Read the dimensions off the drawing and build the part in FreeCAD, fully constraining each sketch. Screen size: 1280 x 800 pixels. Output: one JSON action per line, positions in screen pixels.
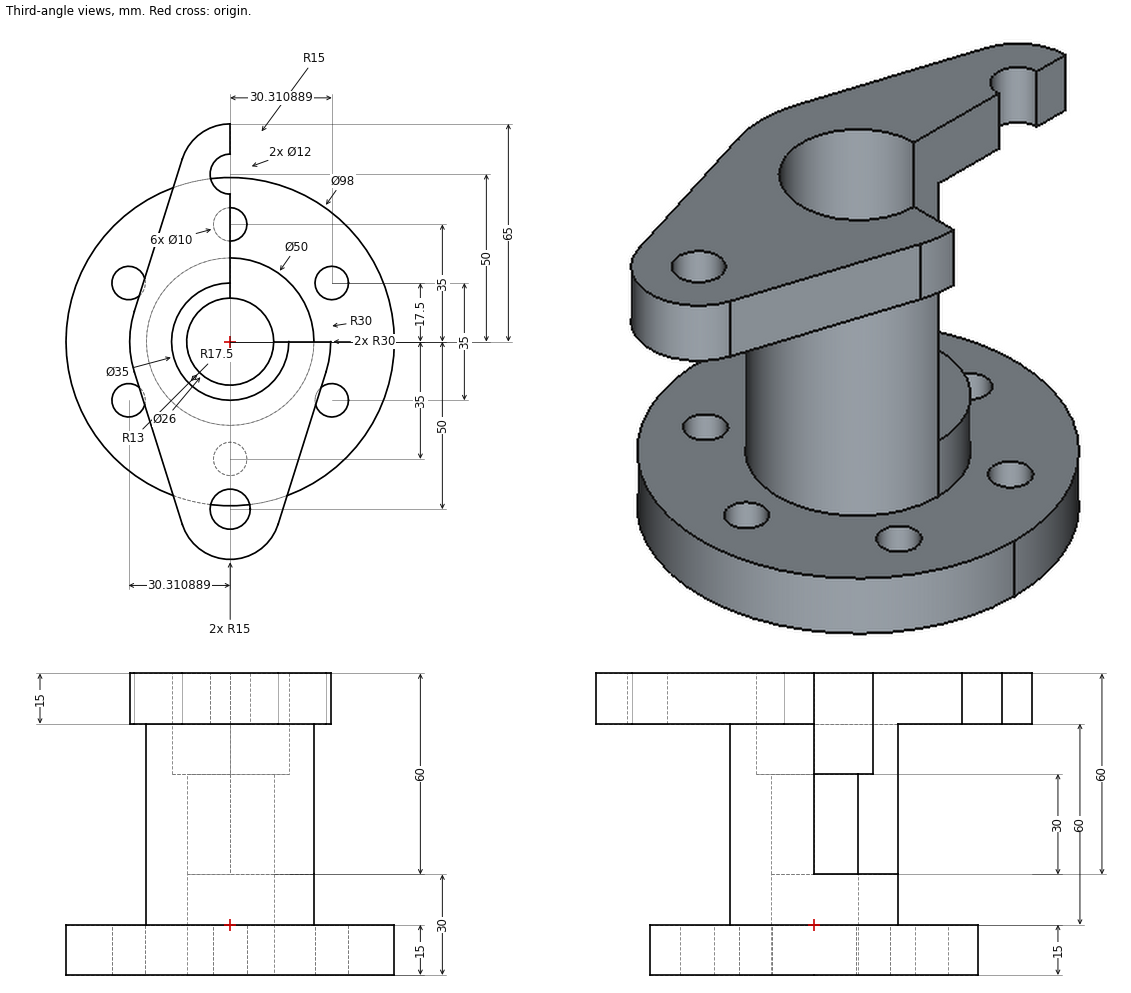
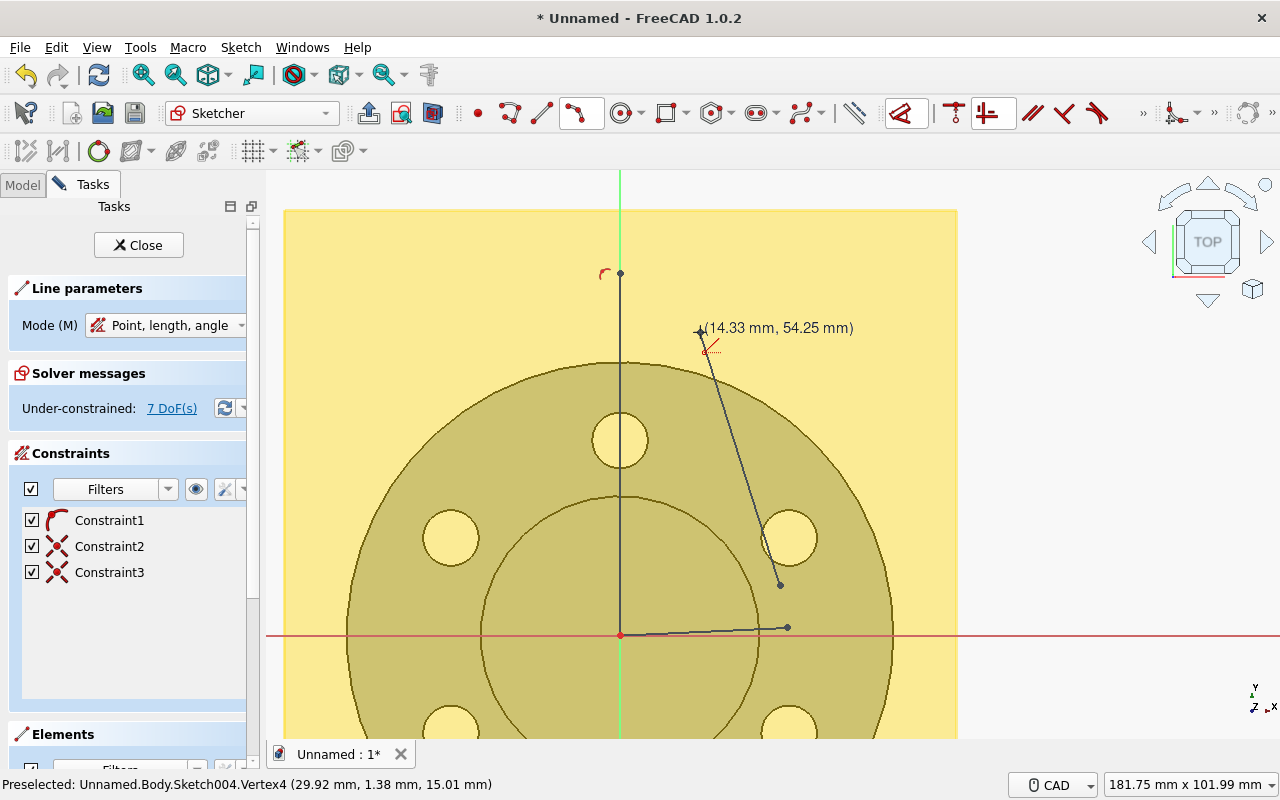
{"action": "left_click", "coordinate": [576, 114]}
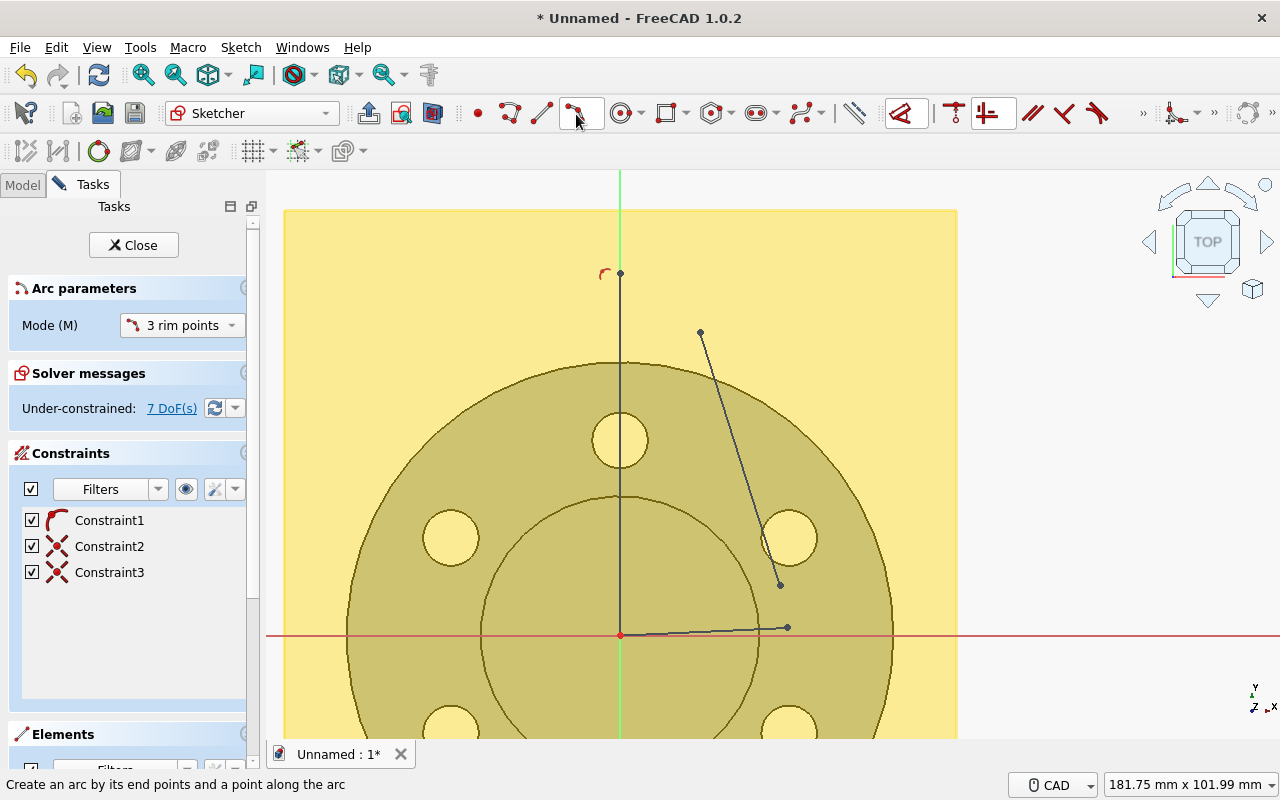
{"action": "left_click", "coordinate": [787, 628]}
{"action": "left_click", "coordinate": [780, 586]}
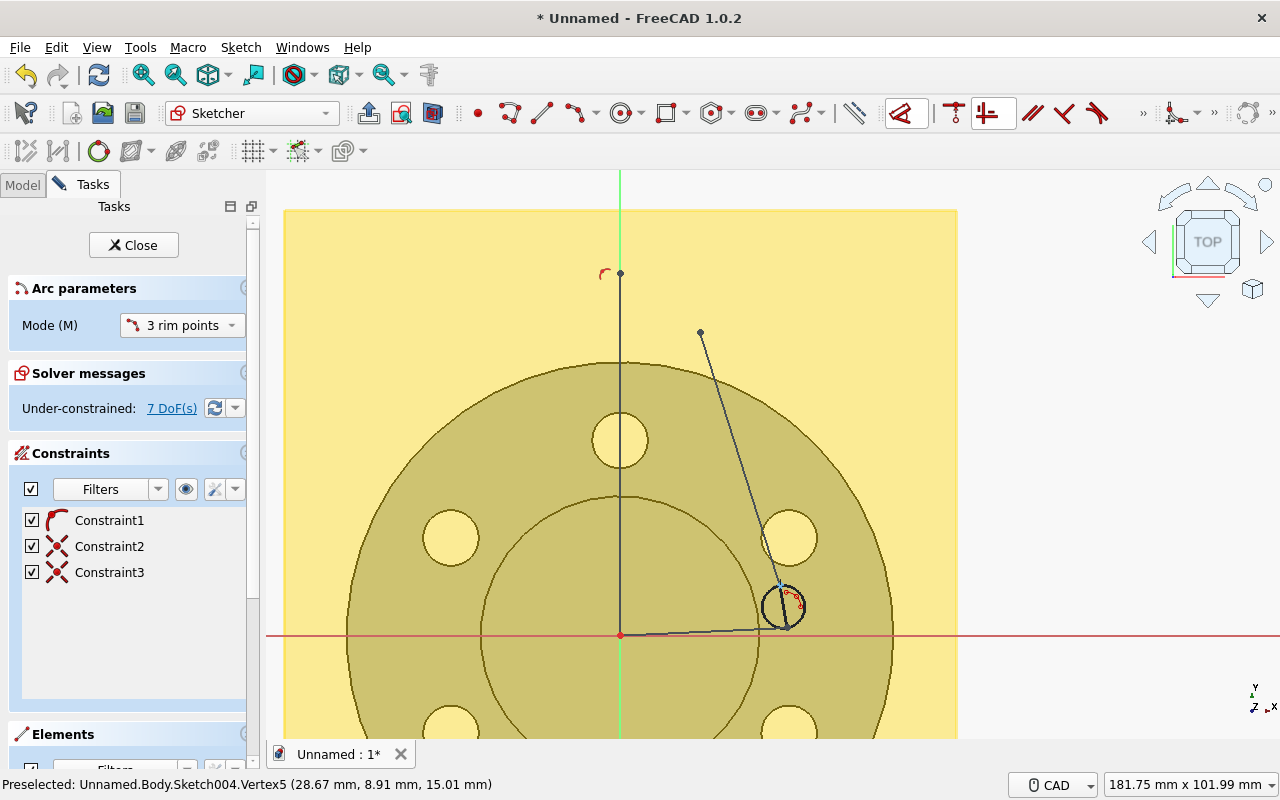
{"action": "scroll", "coordinate": [786, 610], "scroll_direction": "up", "scroll_amount": 11}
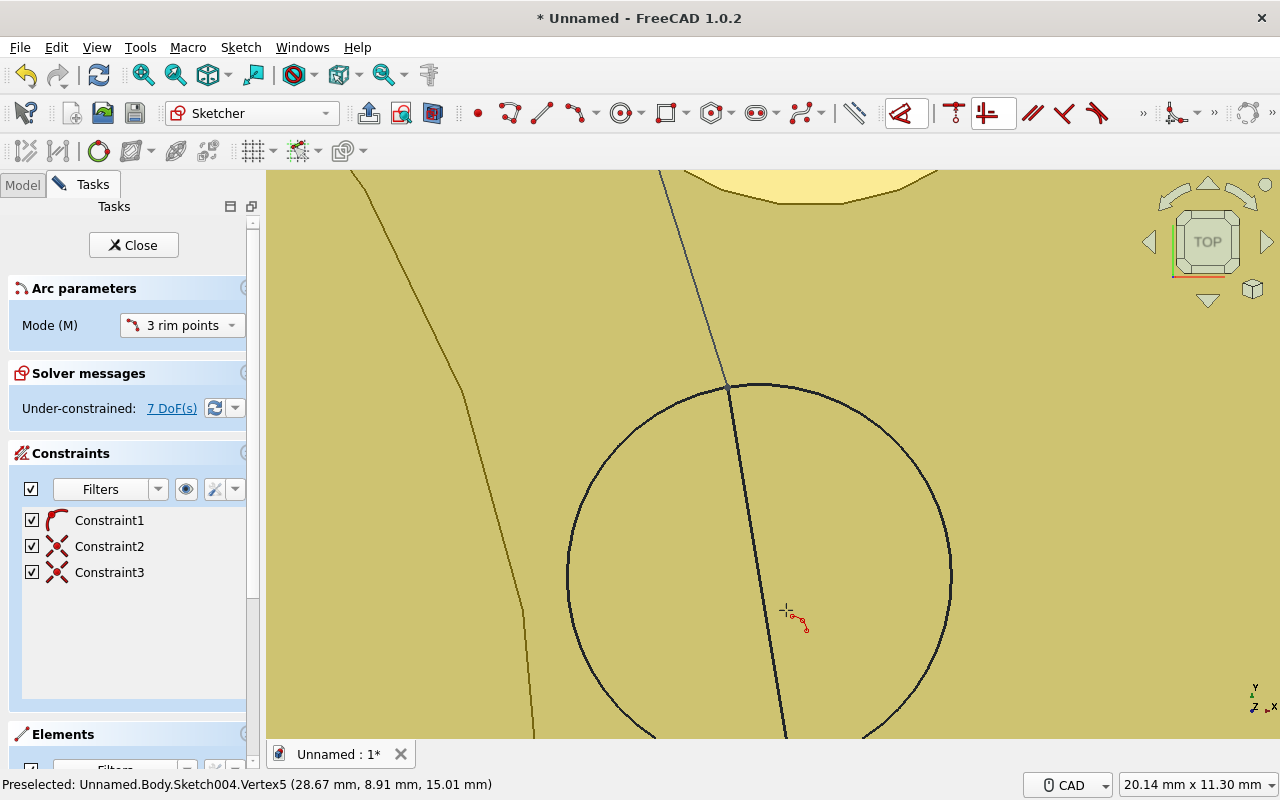
{"action": "left_click", "coordinate": [777, 606]}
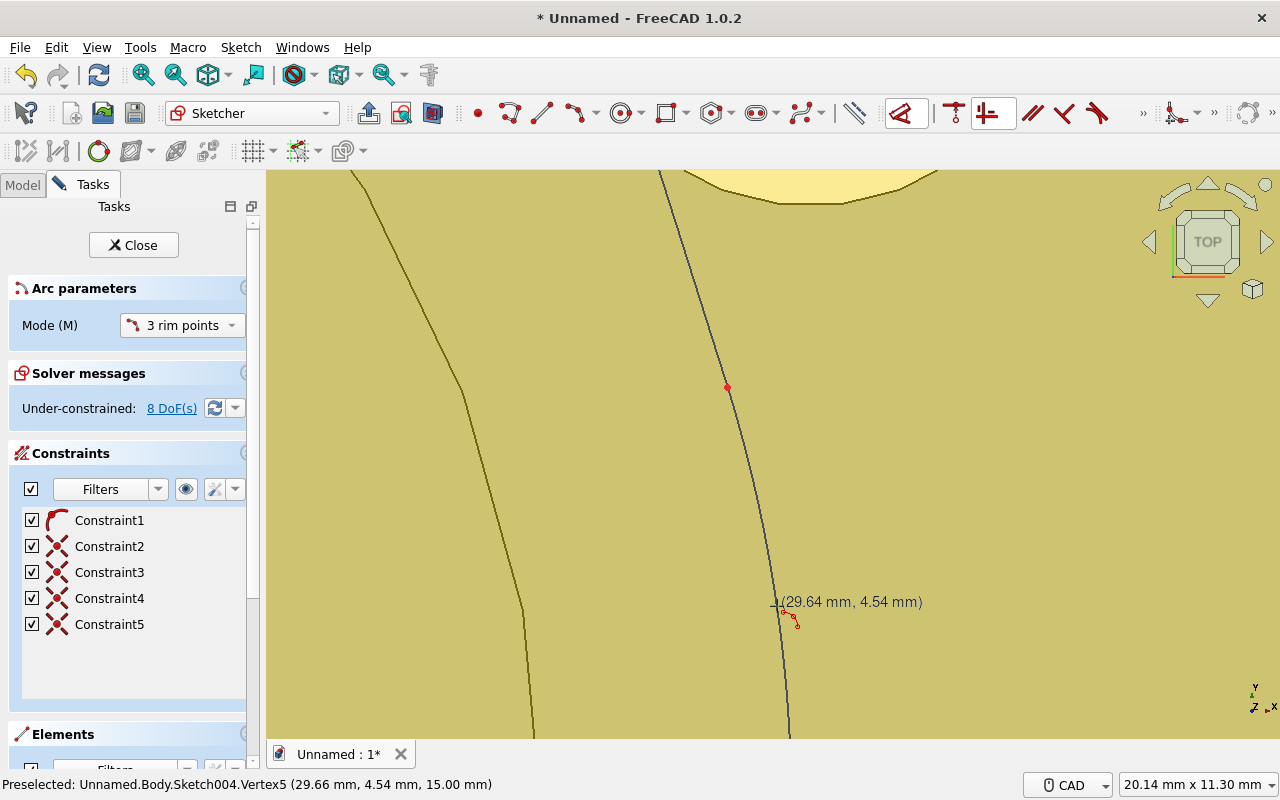
{"action": "scroll", "coordinate": [787, 611], "scroll_direction": "down", "scroll_amount": 11}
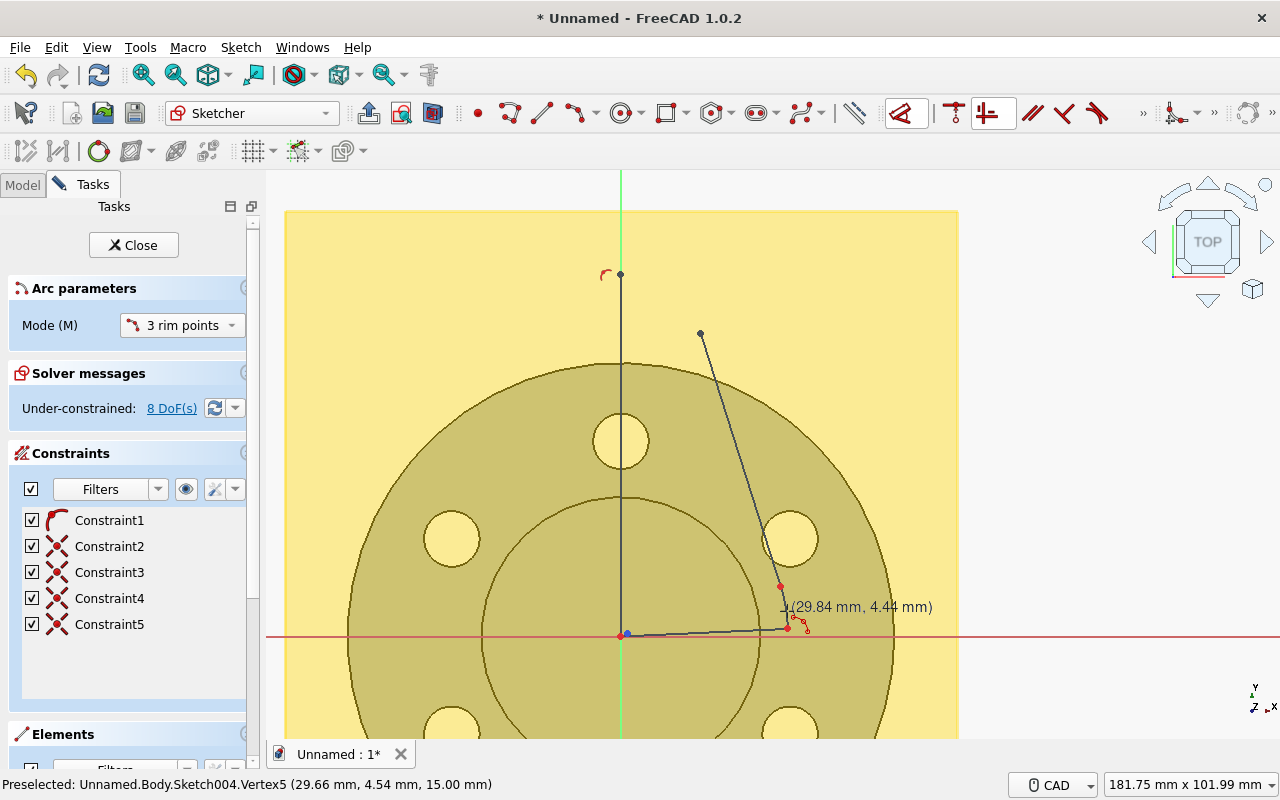
{"action": "left_click", "coordinate": [701, 334]}
{"action": "left_click", "coordinate": [621, 275]}
{"action": "left_click", "coordinate": [670, 290]}
{"action": "key", "text": "Escape"}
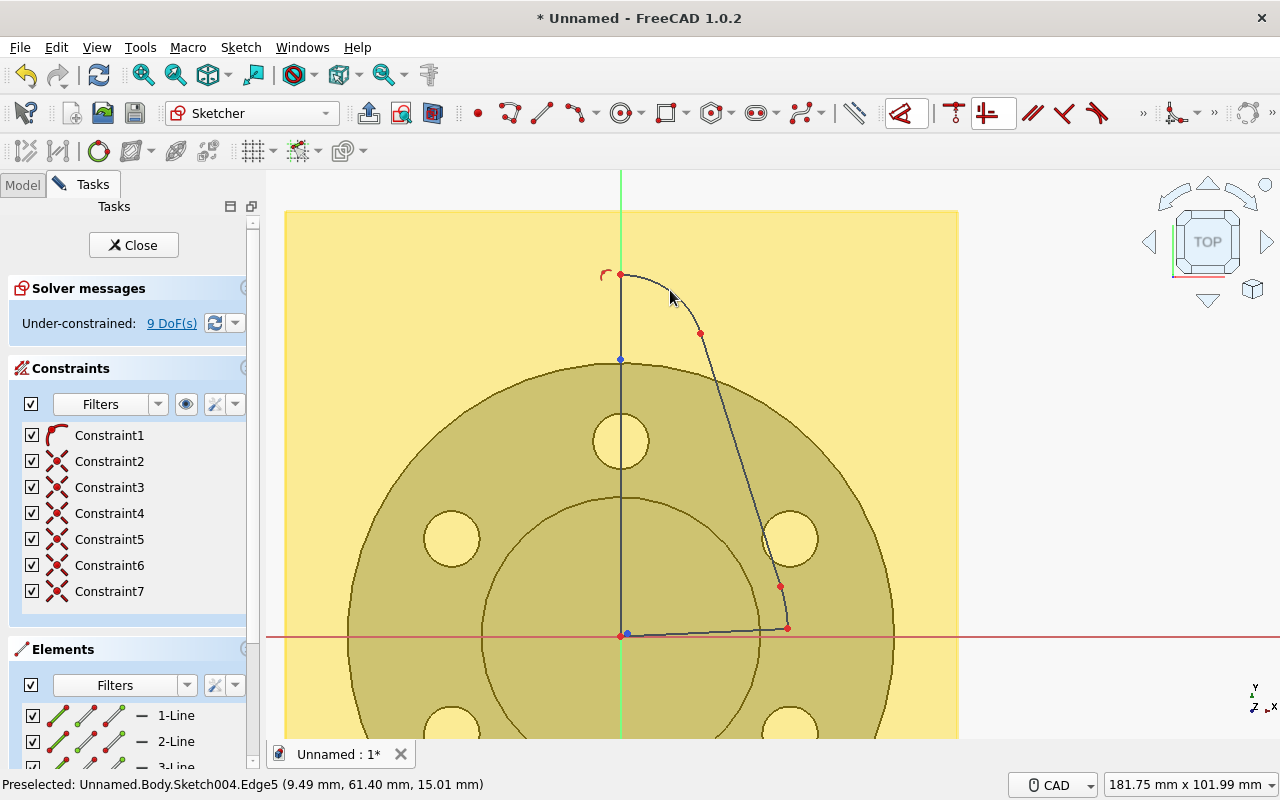
{"action": "left_click", "coordinate": [757, 511]}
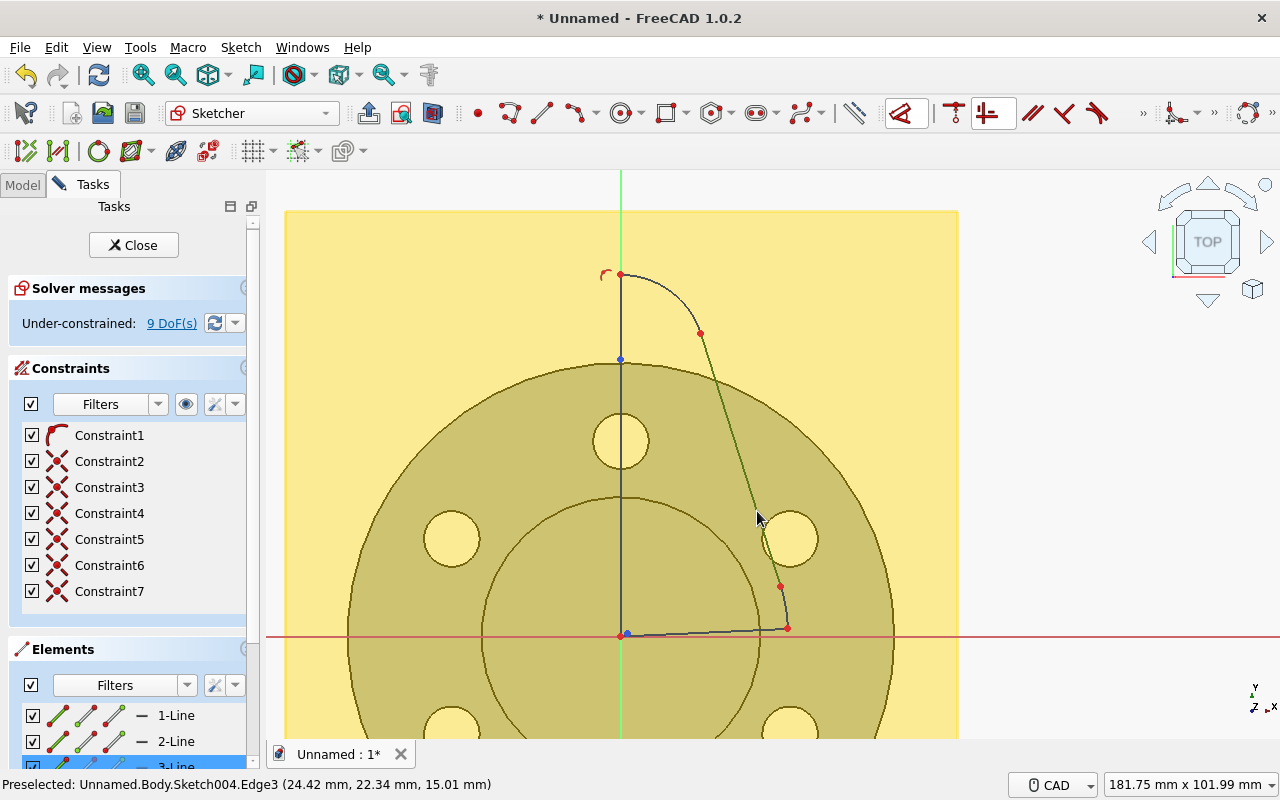
{"action": "left_click", "coordinate": [787, 616]}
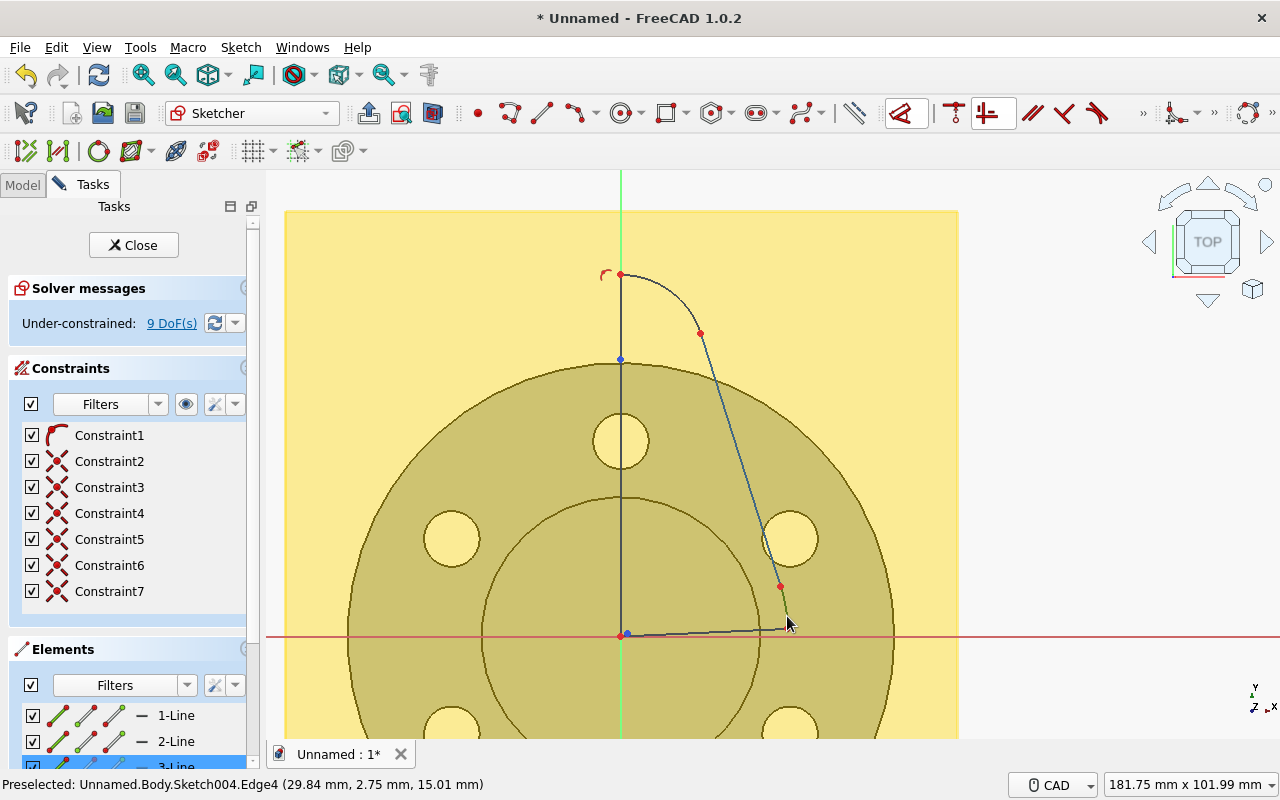
{"action": "key", "text": "t"}